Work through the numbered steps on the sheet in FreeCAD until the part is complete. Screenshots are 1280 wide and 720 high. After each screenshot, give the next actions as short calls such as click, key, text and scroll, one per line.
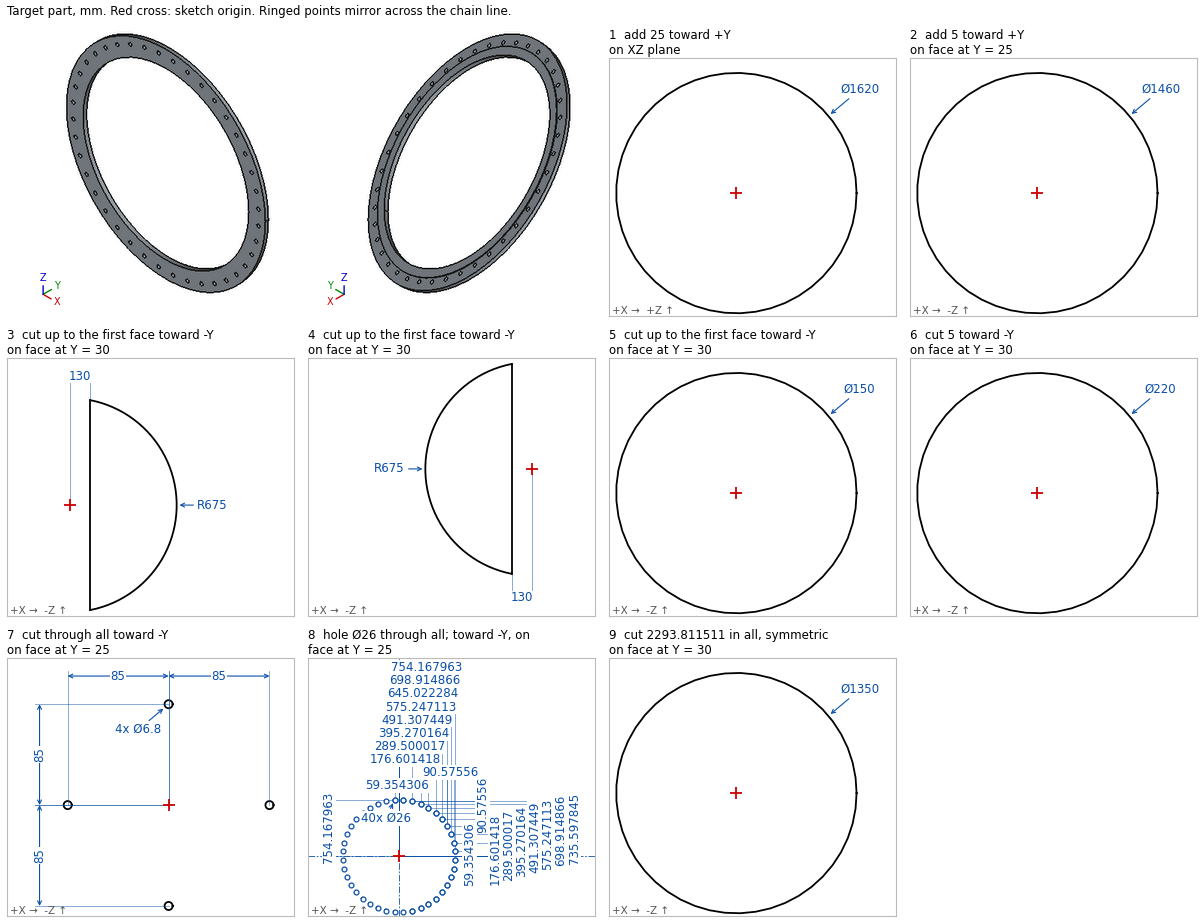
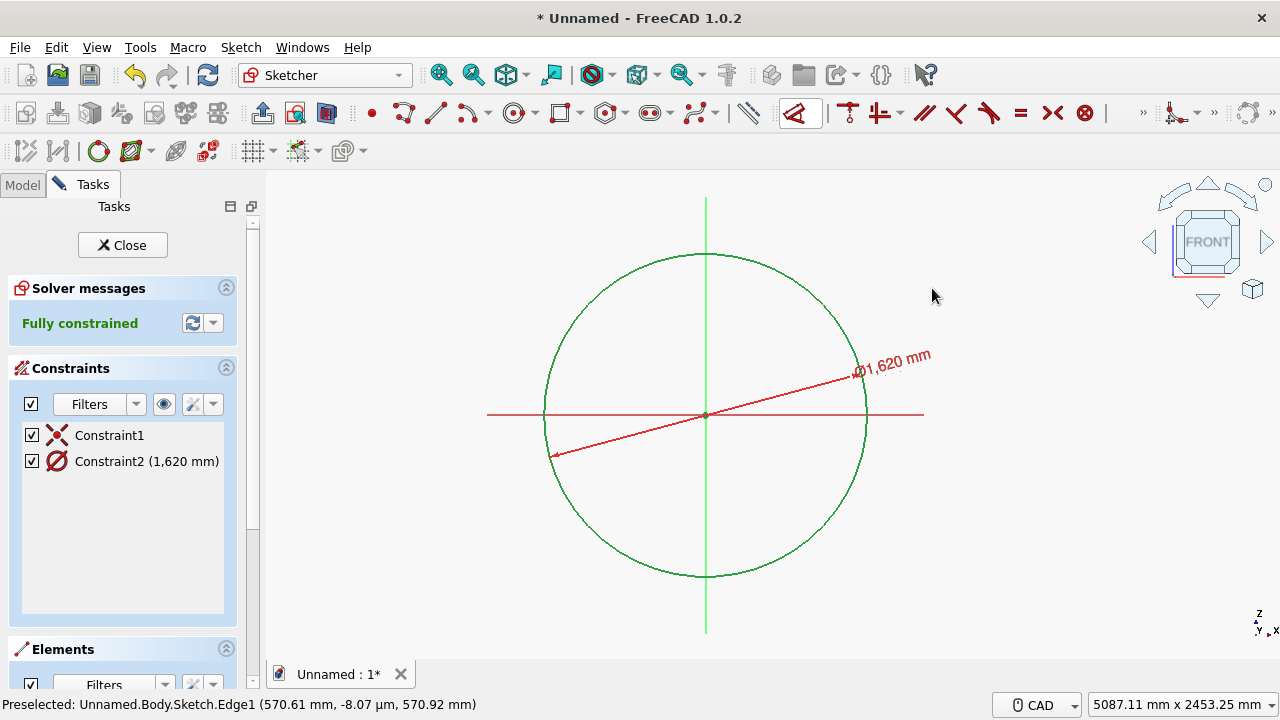
click(123, 245)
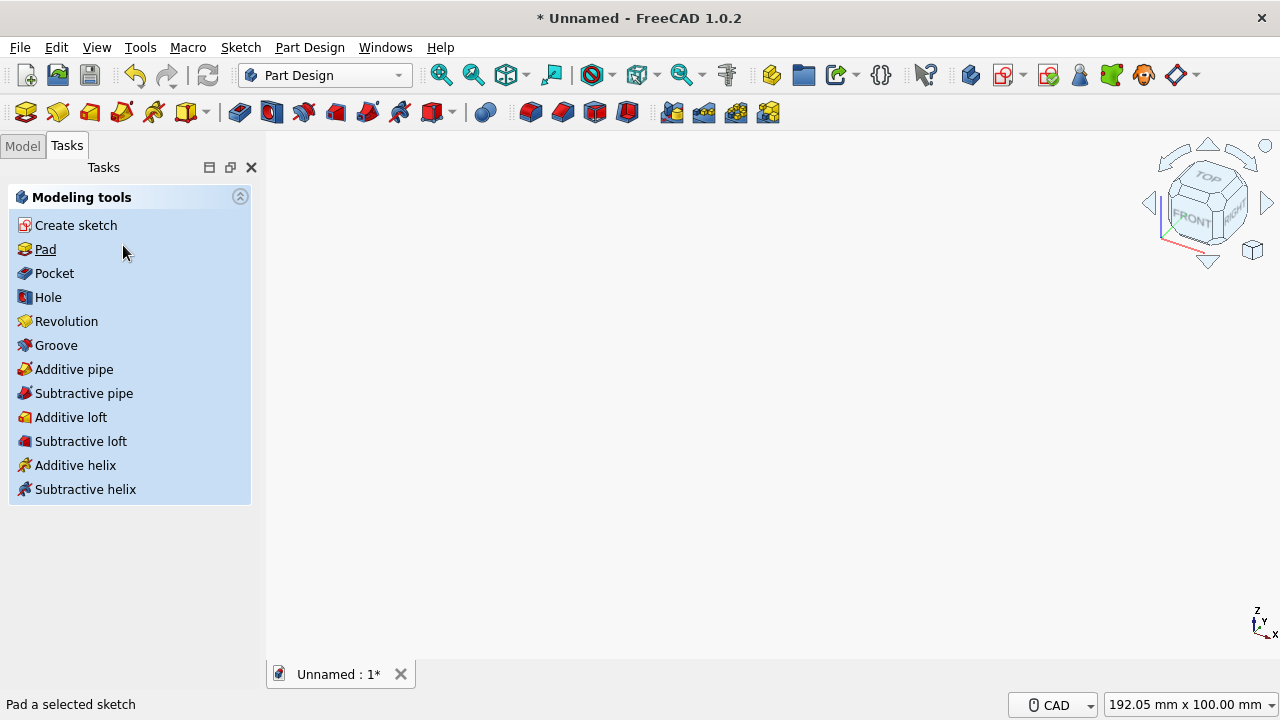
click(26, 112)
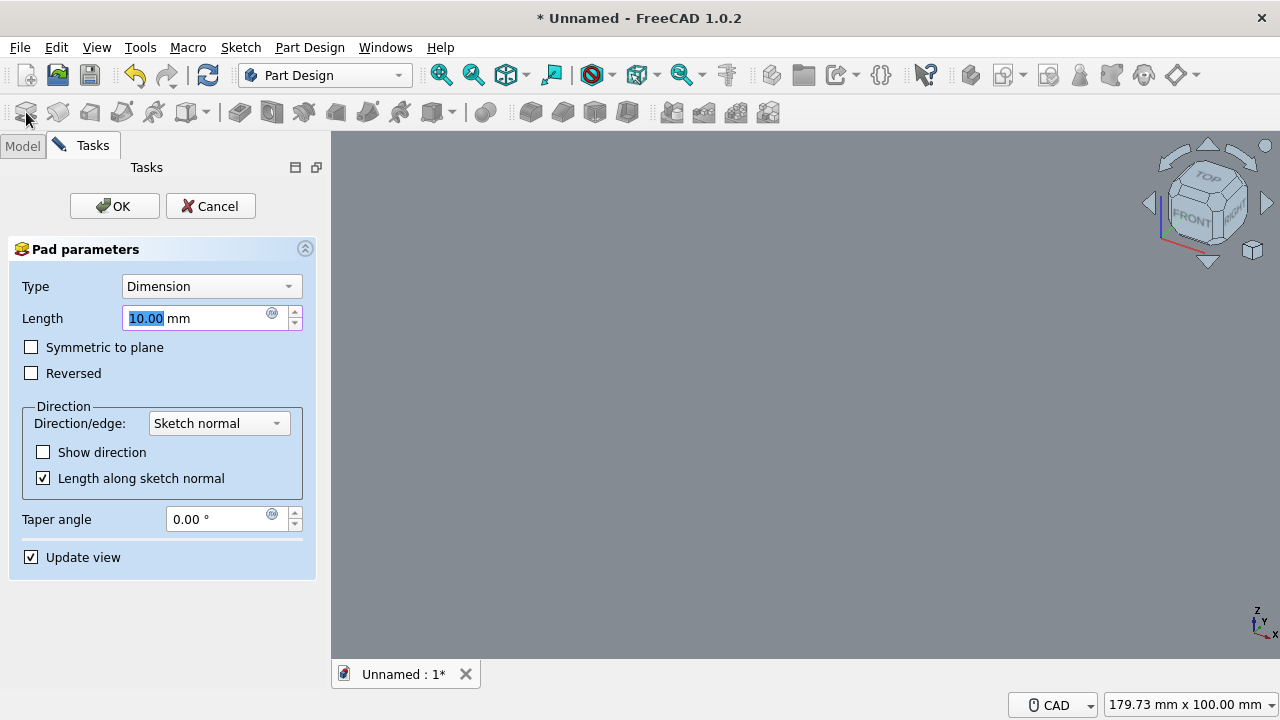
text(25)
key(Tab)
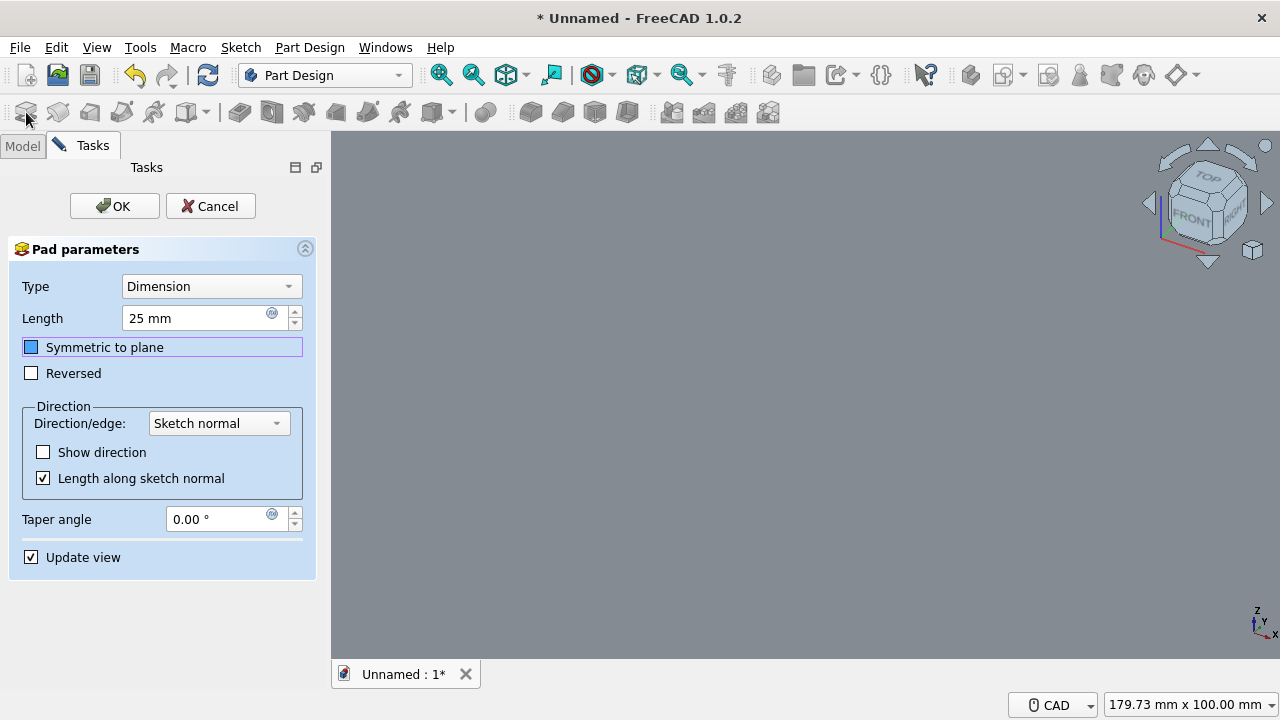
click(30, 373)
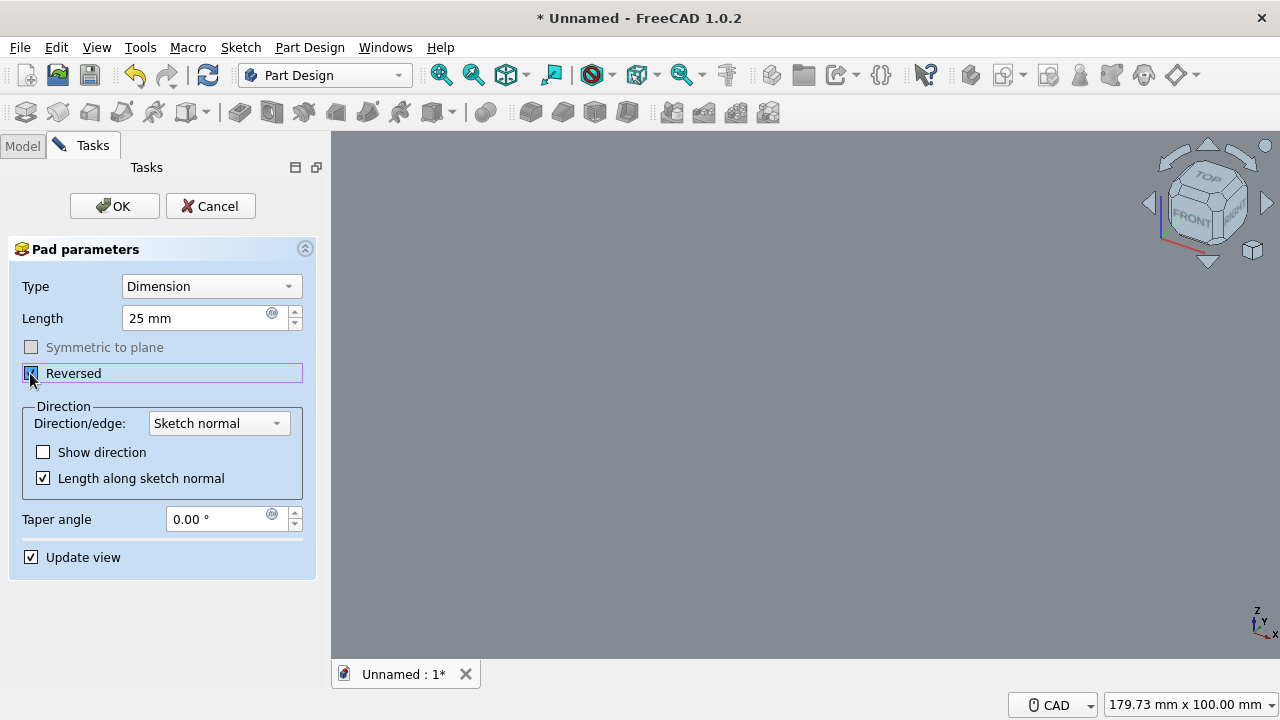
click(115, 206)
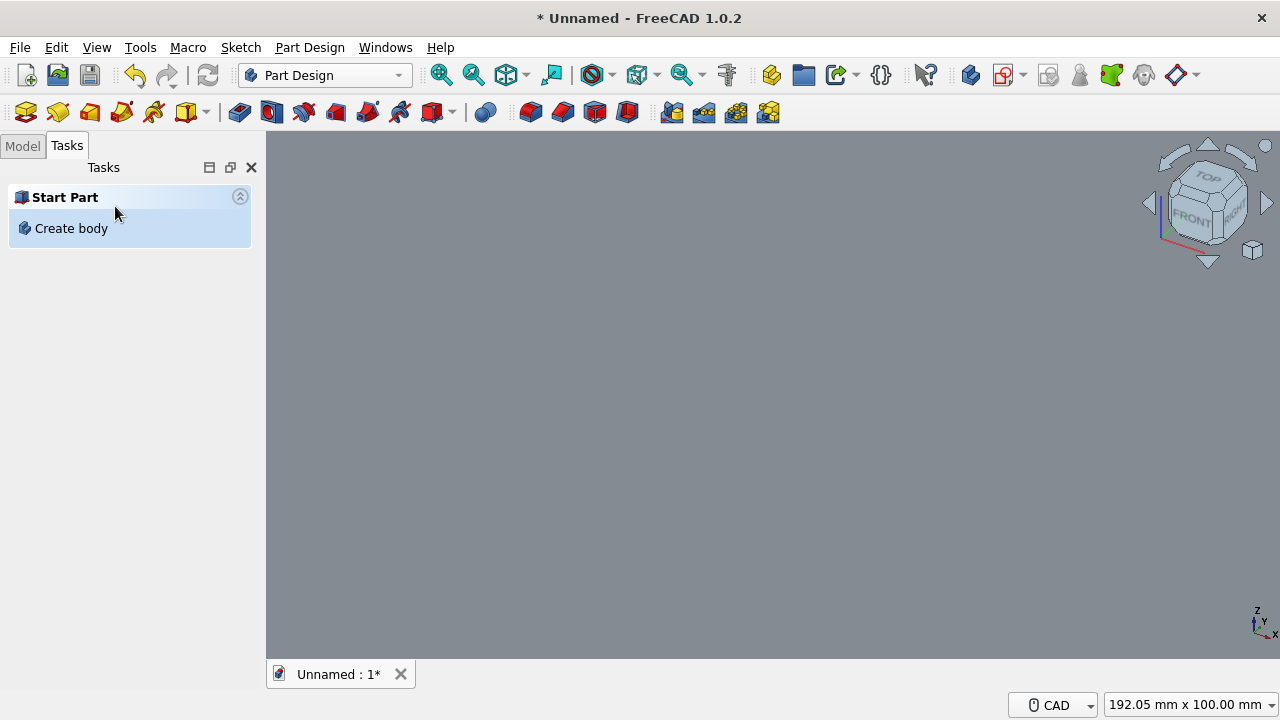
click(442, 76)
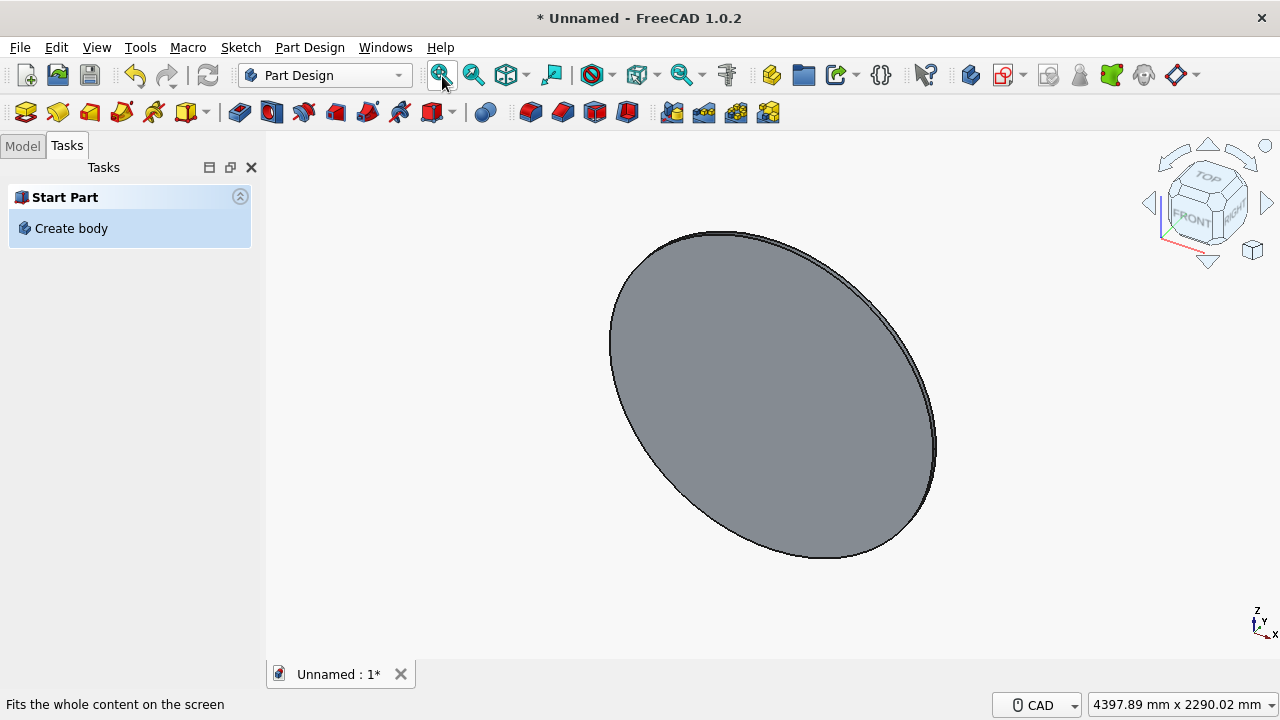
key(4)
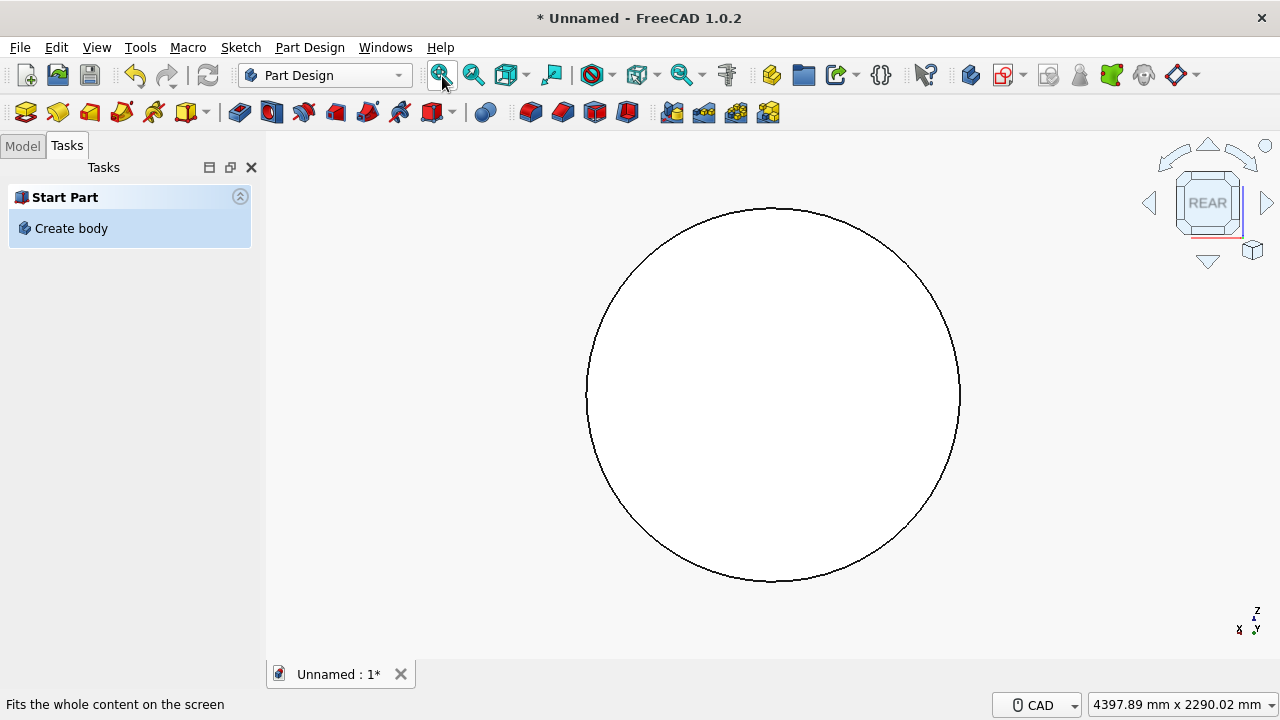
click(773, 394)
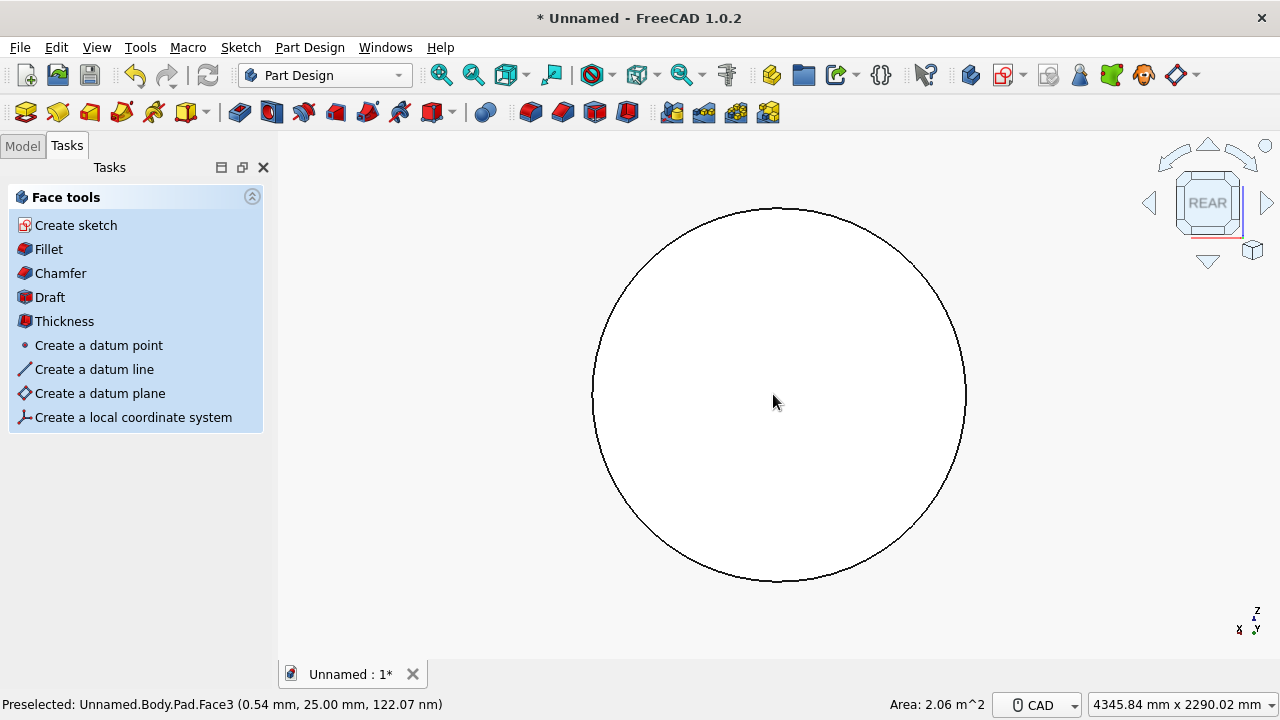
click(1004, 76)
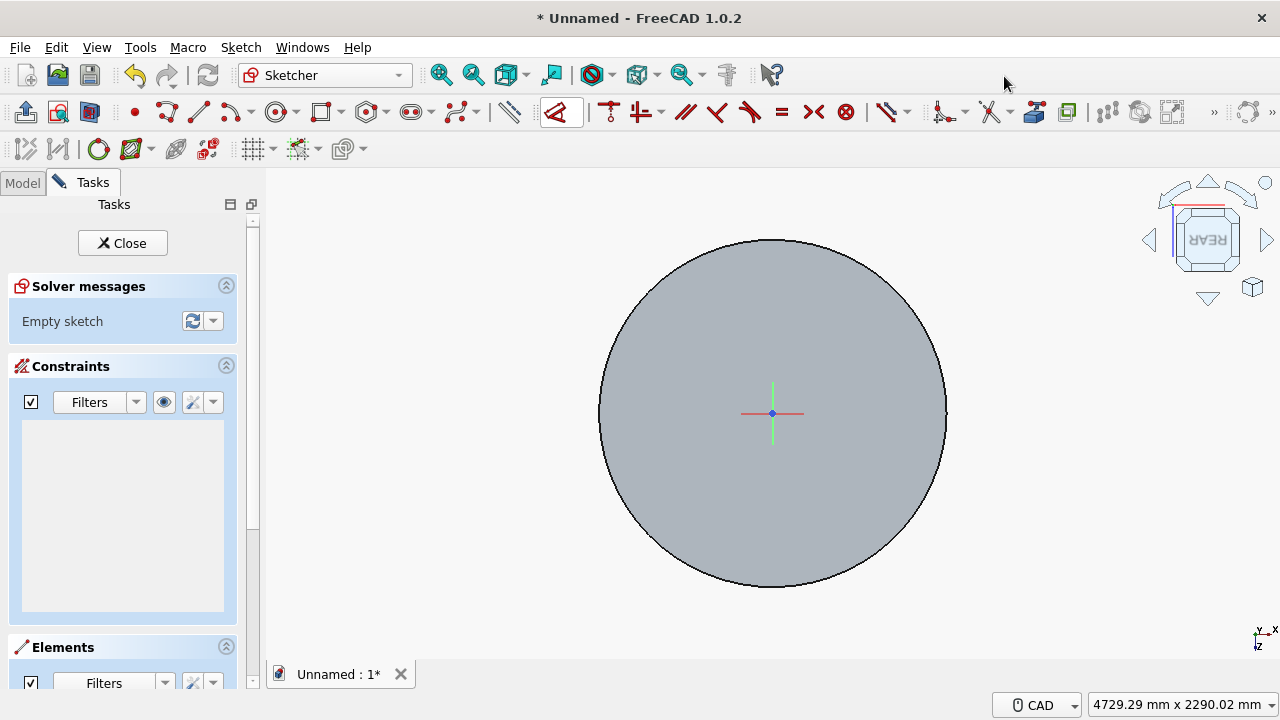
click(276, 112)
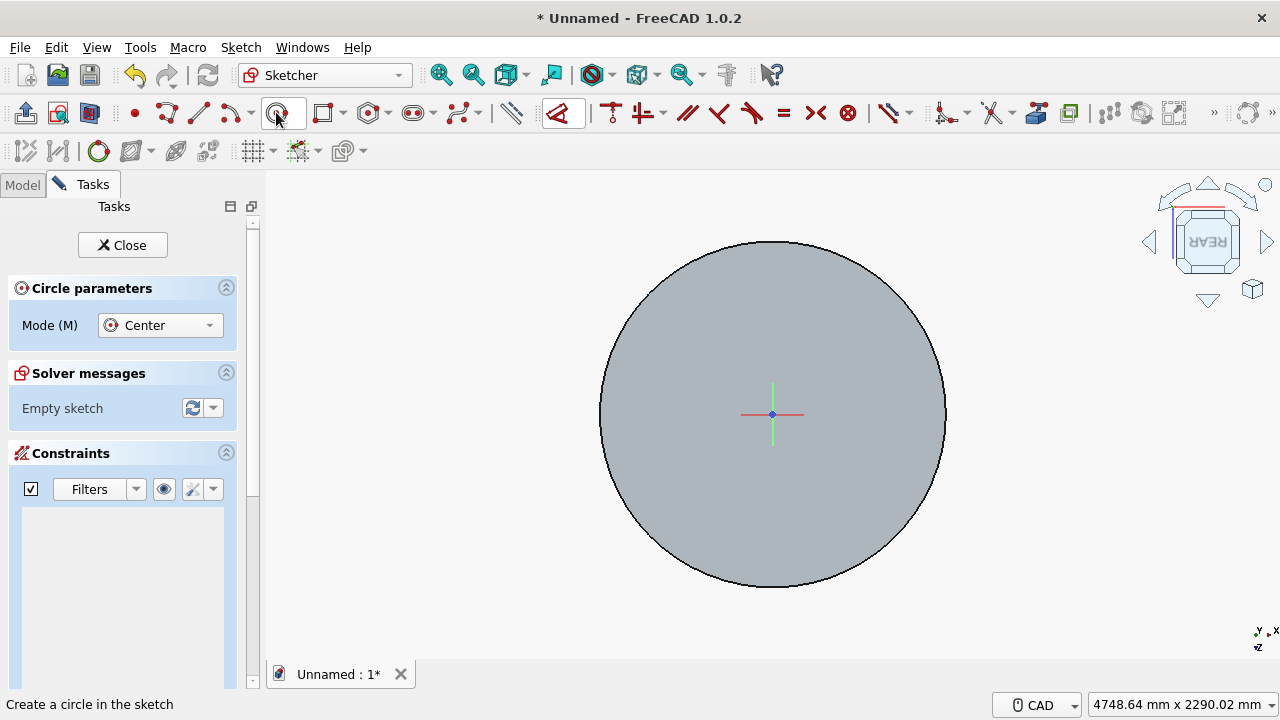
click(773, 414)
click(883, 304)
key(Escape)